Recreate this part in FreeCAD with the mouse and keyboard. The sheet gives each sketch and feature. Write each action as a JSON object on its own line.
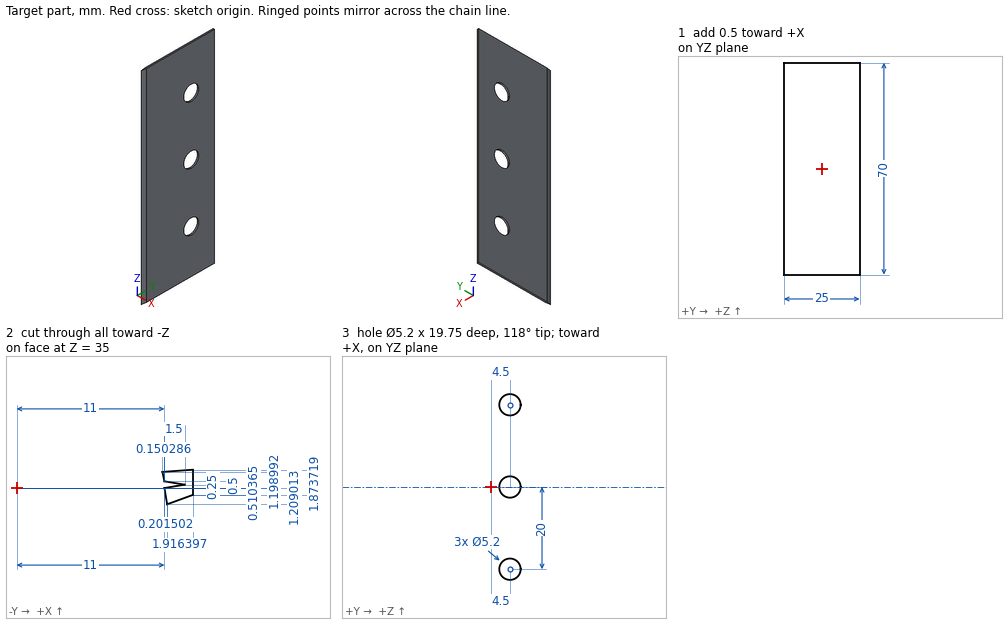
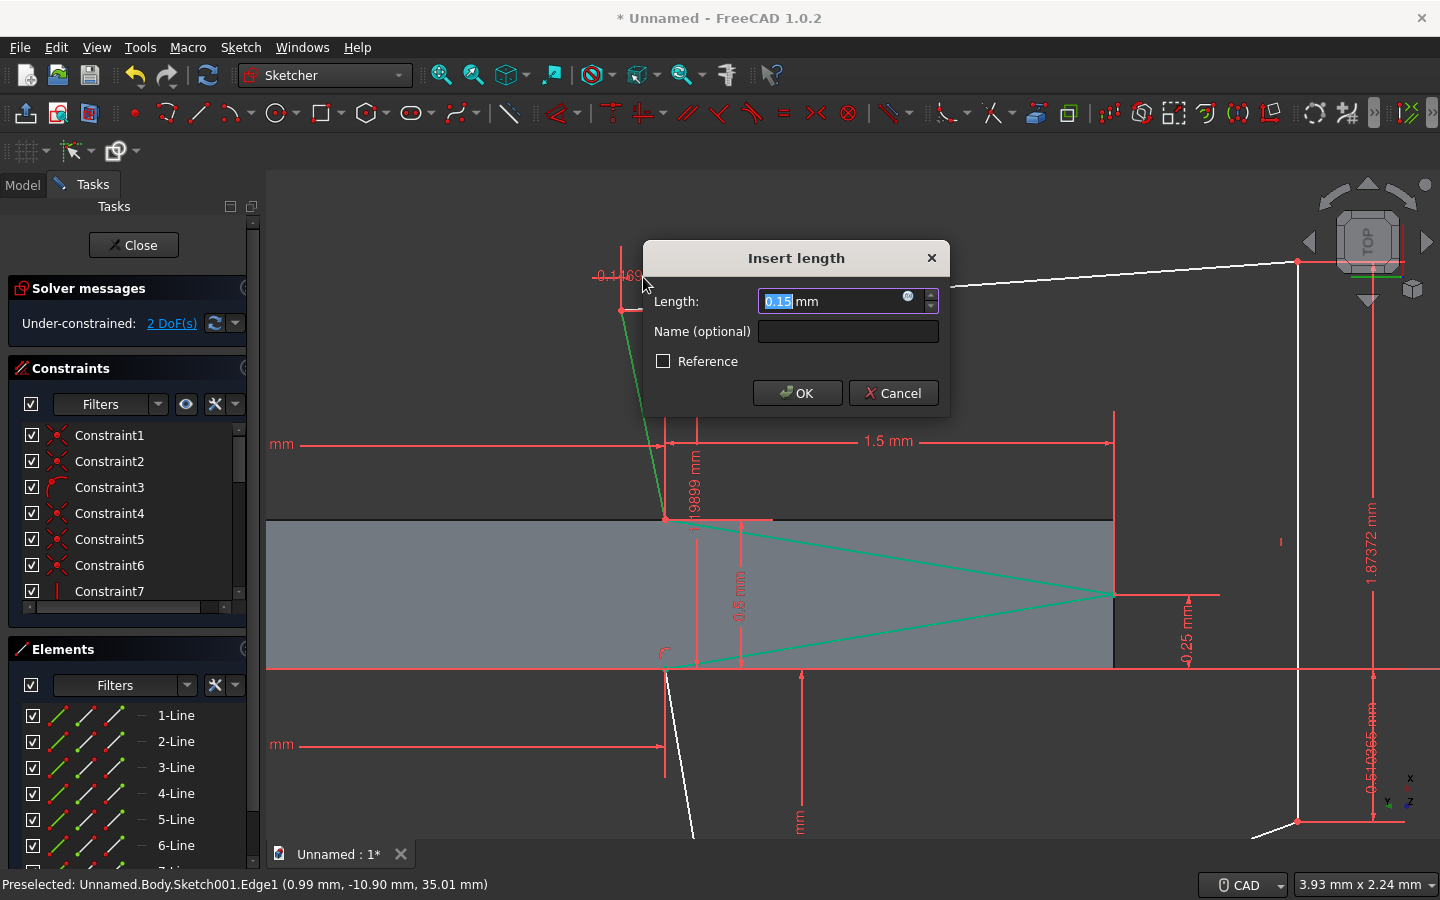
{"action": "type", "text": "0.150286"}
{"action": "key", "text": "Return"}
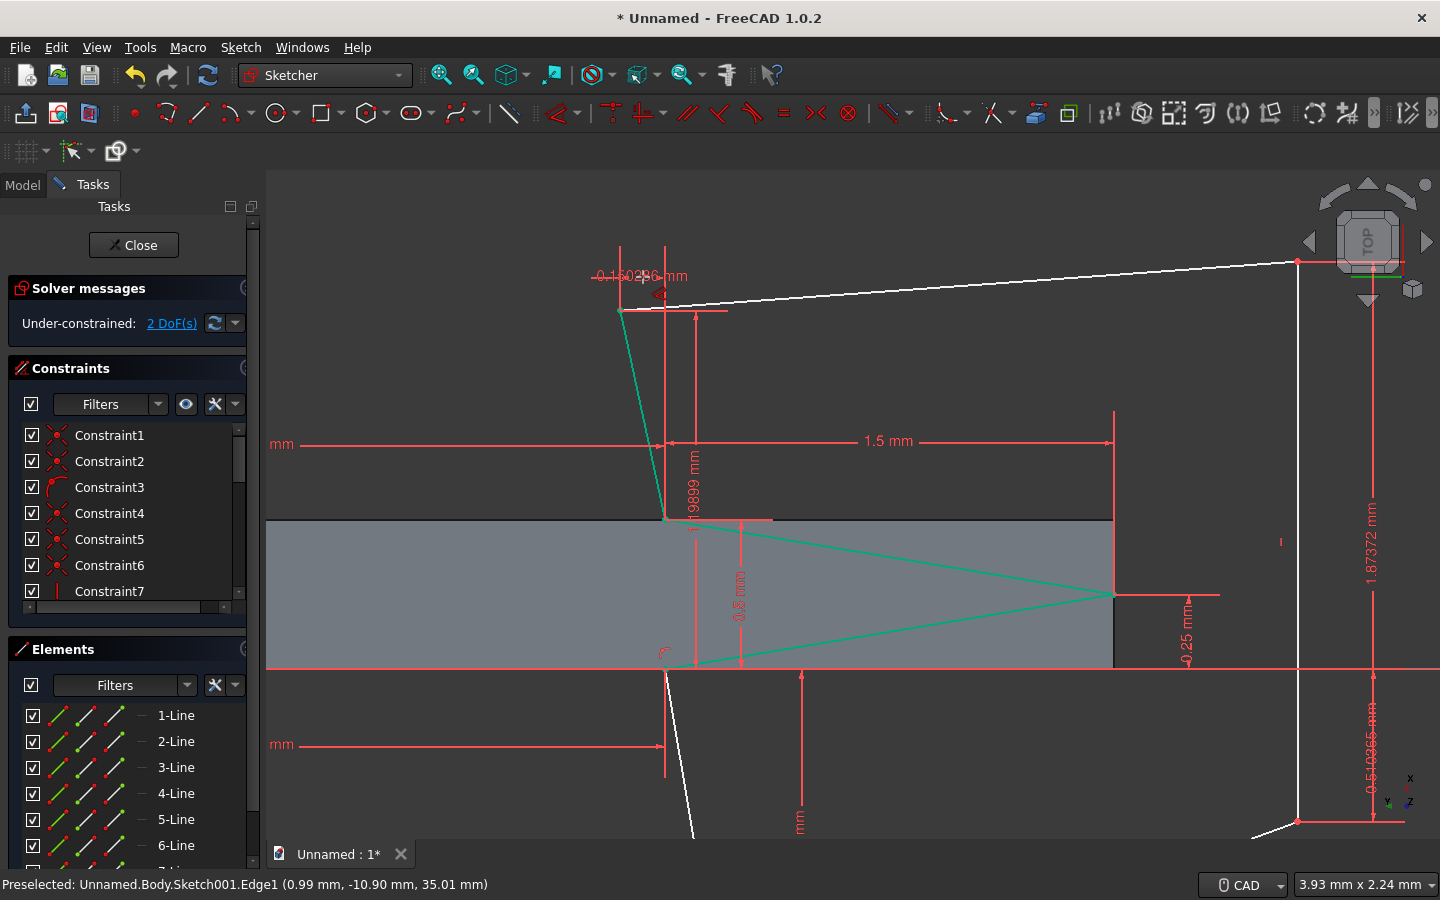
{"action": "left_click", "coordinate": [683, 778]}
{"action": "left_click", "coordinate": [696, 635]}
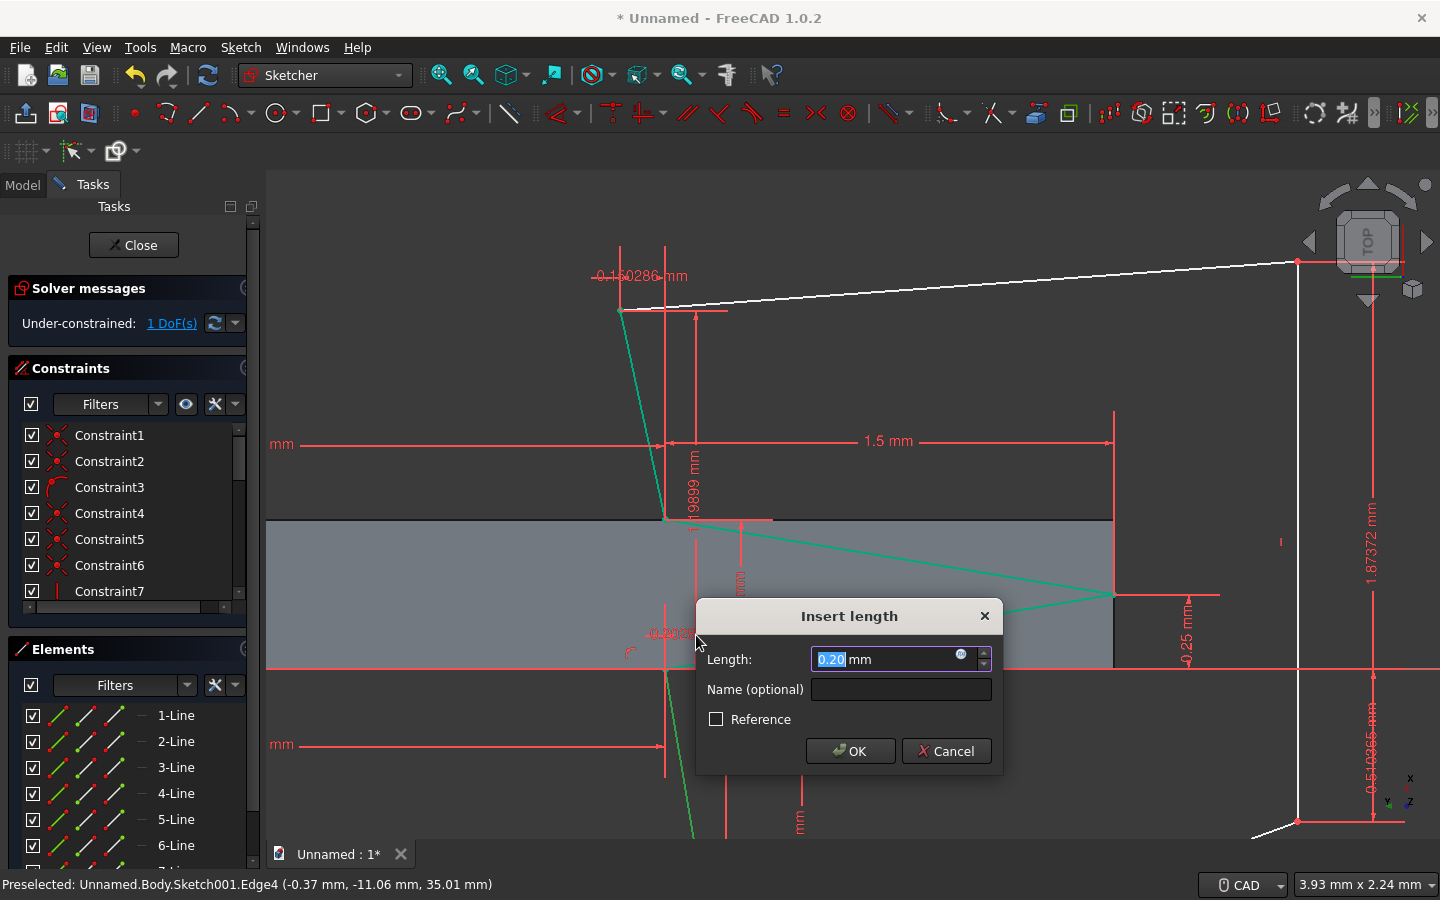
{"action": "type", "text": "0.201502"}
{"action": "key", "text": "Return"}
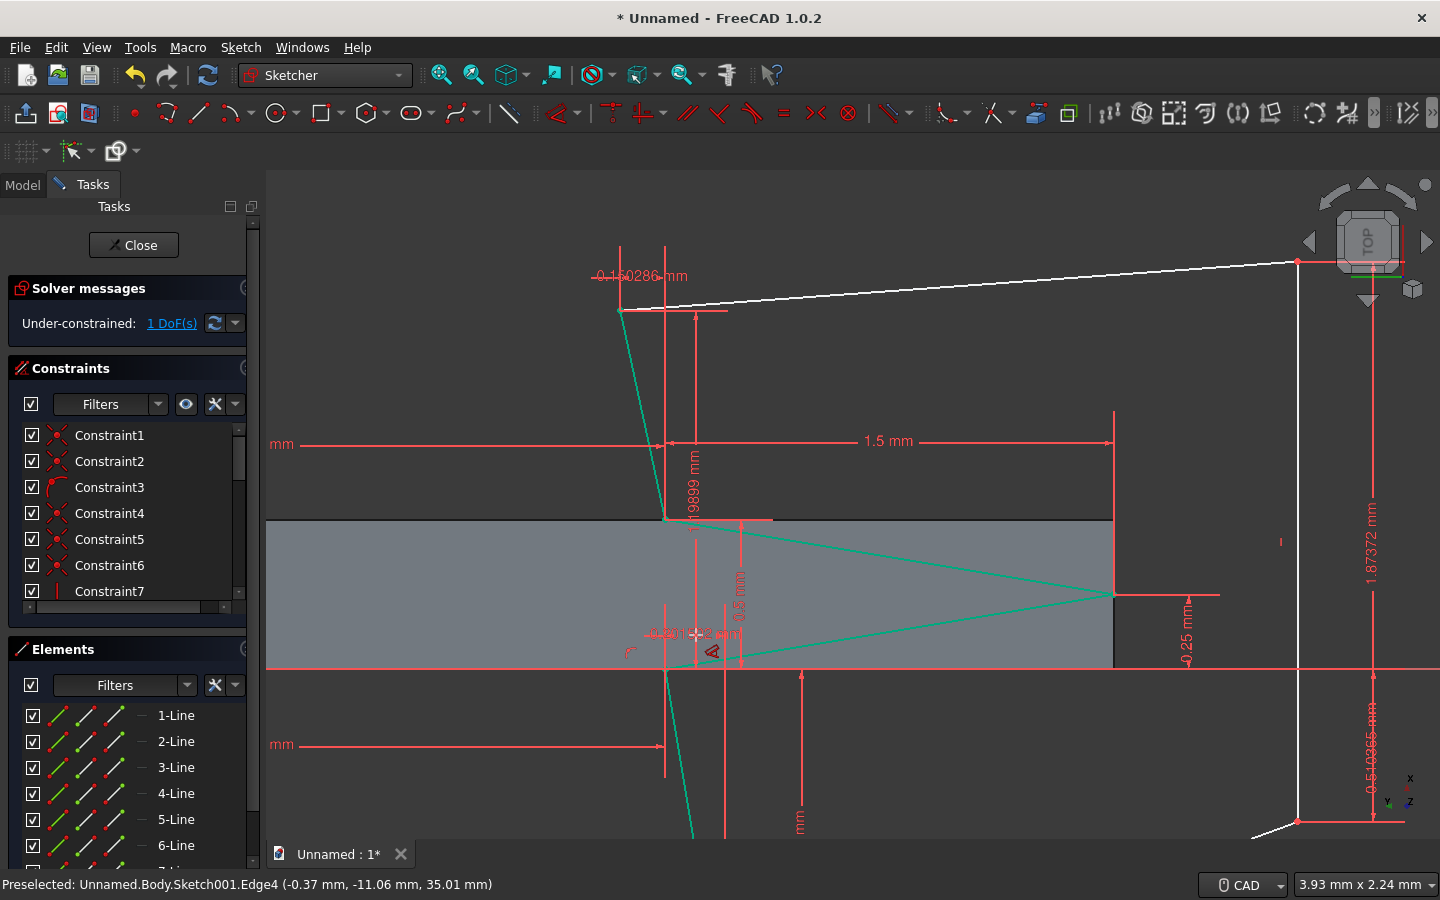
{"action": "scroll", "coordinate": [572, 332], "scroll_direction": "down", "scroll_amount": 3}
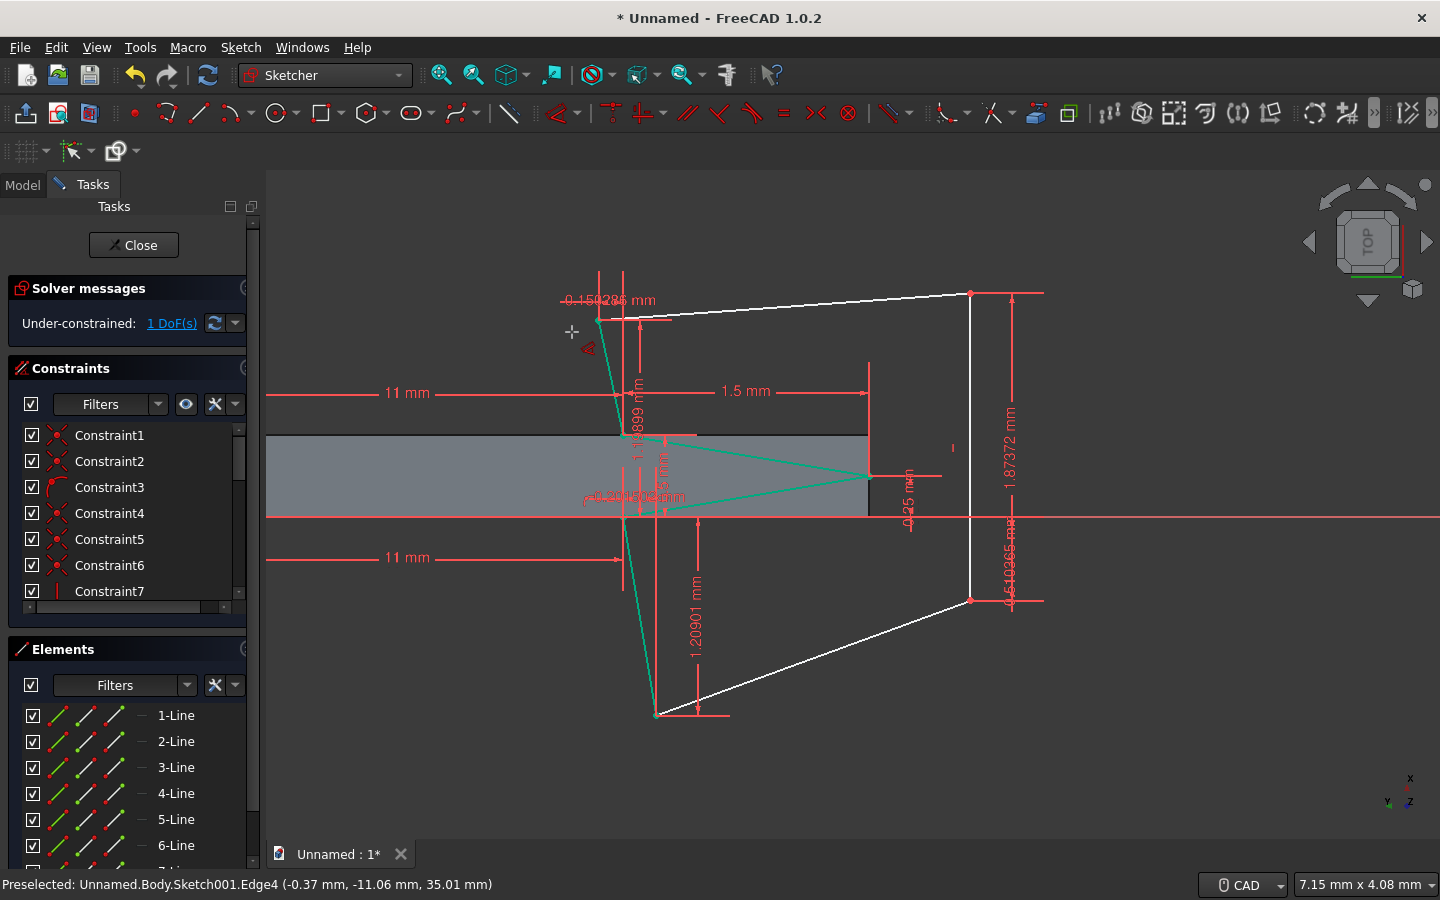
{"action": "left_click", "coordinate": [751, 681]}
{"action": "left_click", "coordinate": [813, 750]}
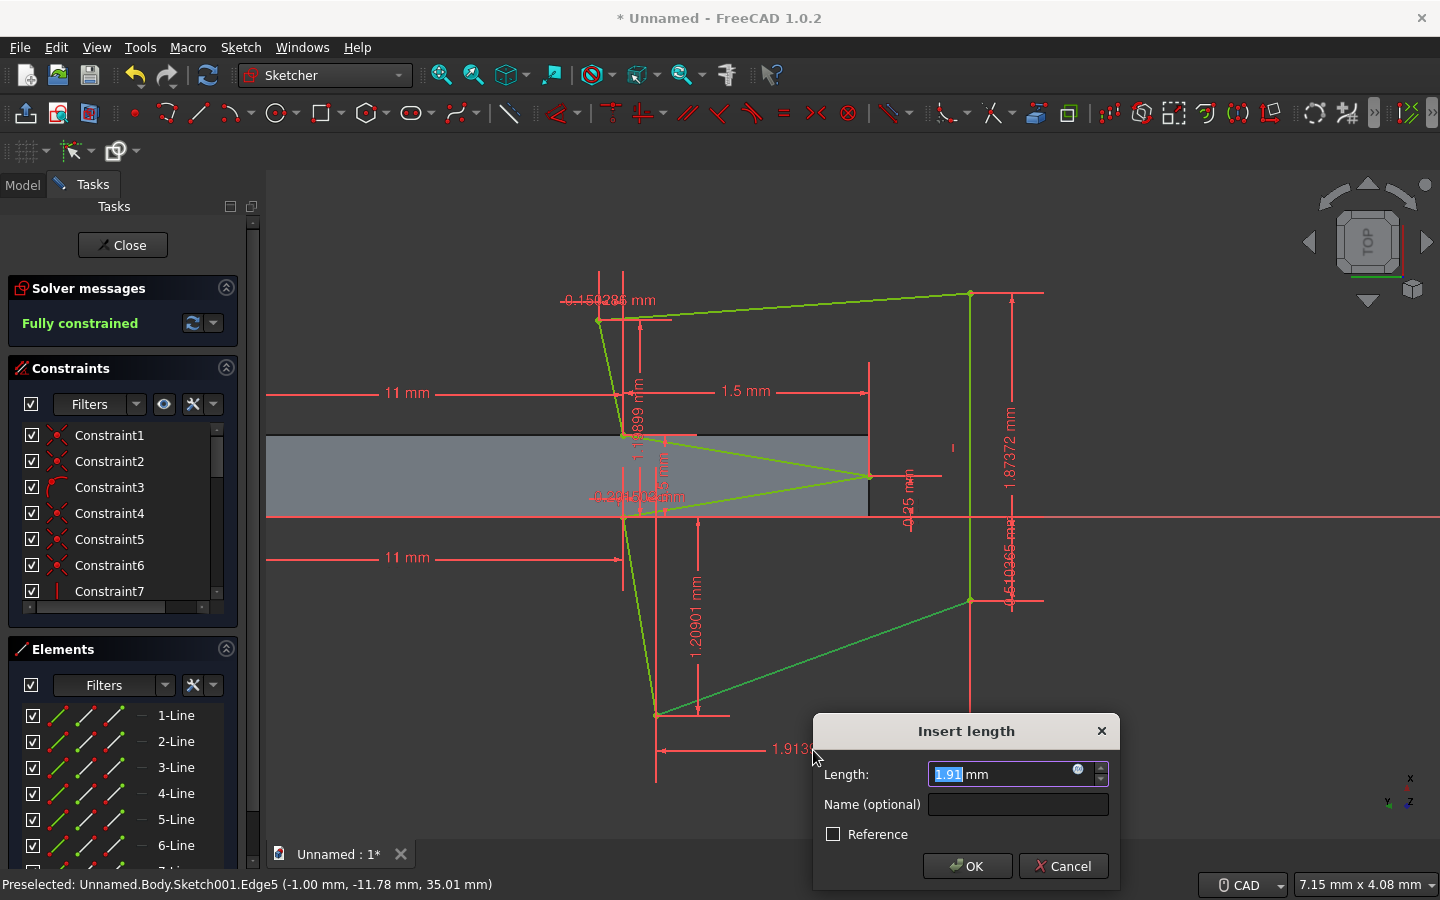
{"action": "type", "text": "1.916397"}
{"action": "key", "text": "Return"}
{"action": "key", "text": "Escape"}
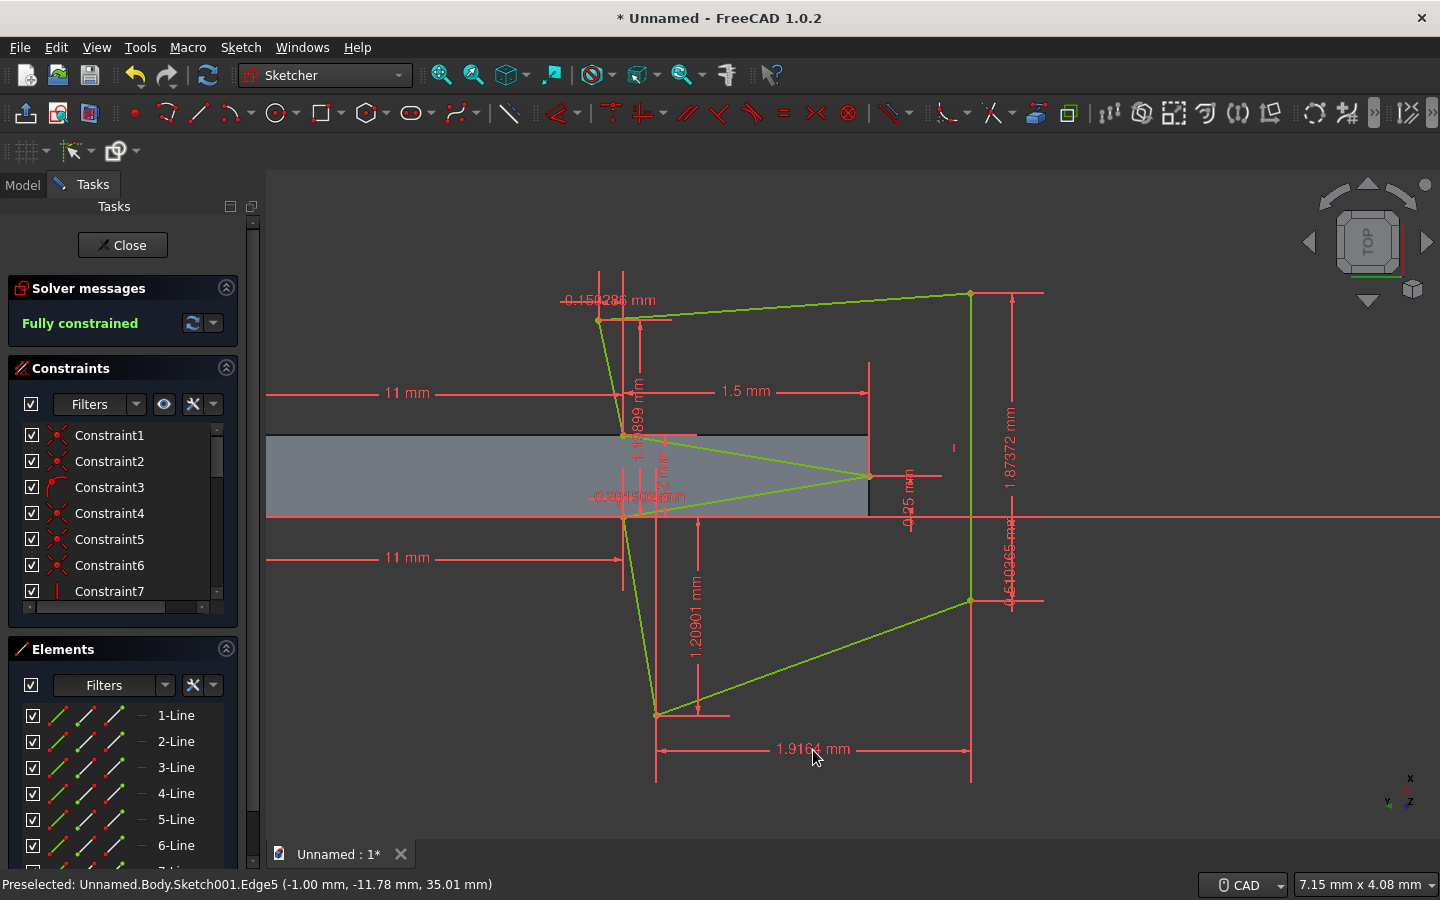
{"action": "left_click", "coordinate": [123, 245]}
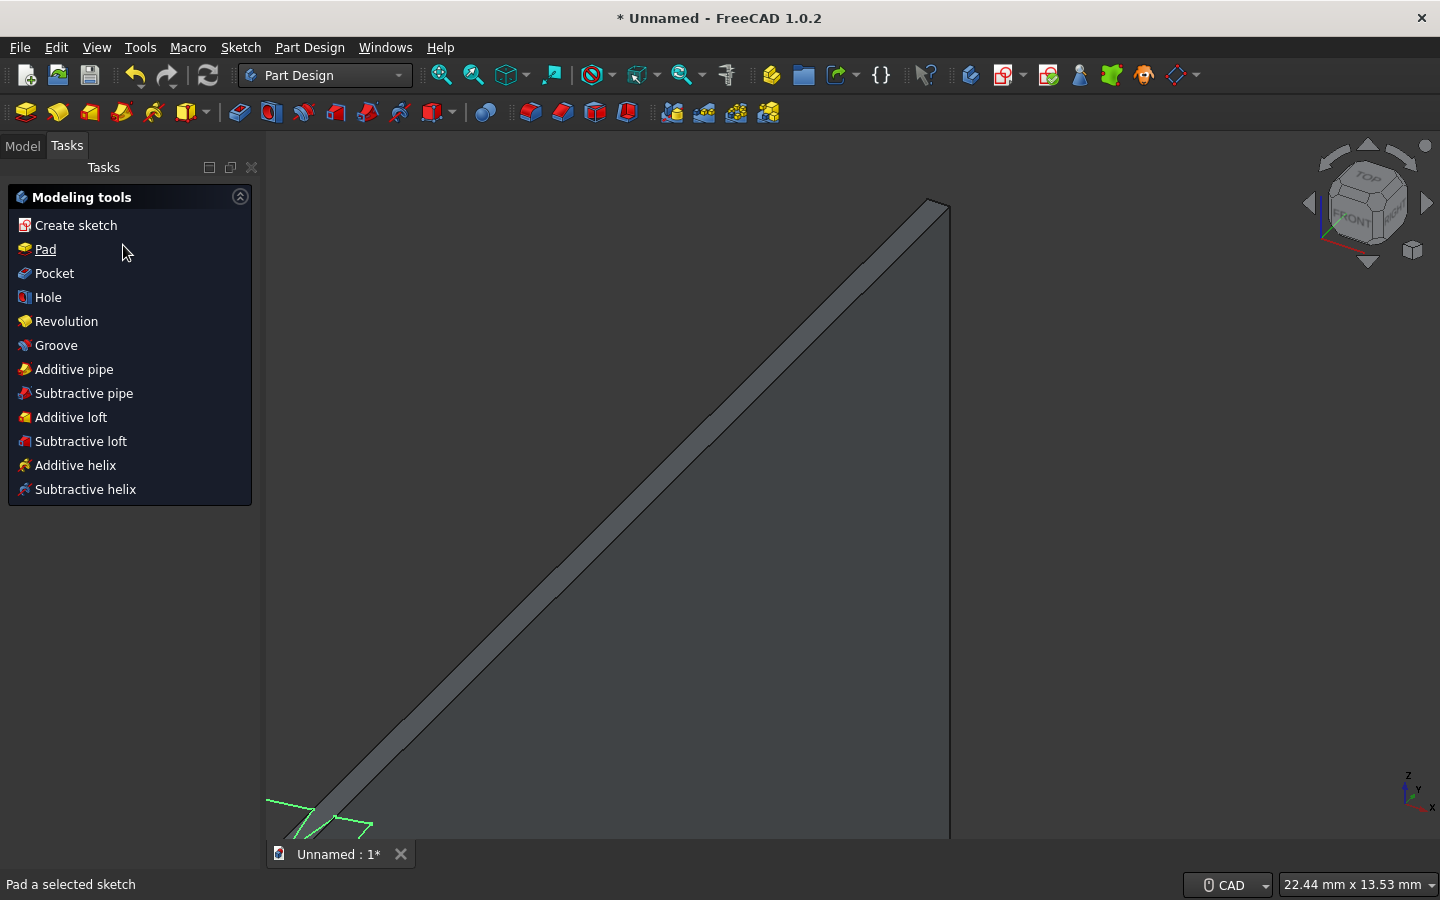
{"action": "left_click", "coordinate": [240, 112]}